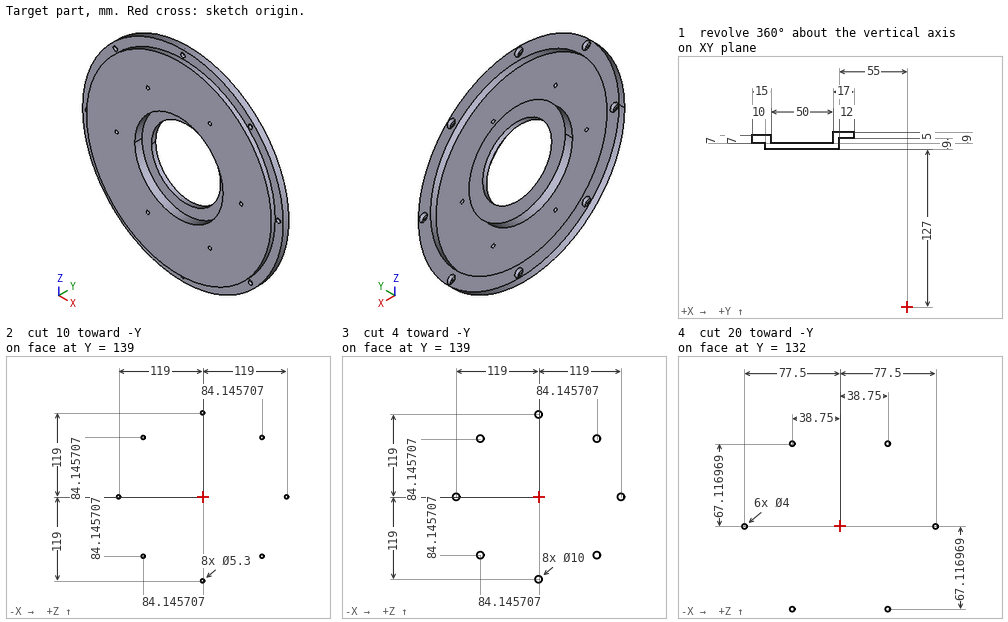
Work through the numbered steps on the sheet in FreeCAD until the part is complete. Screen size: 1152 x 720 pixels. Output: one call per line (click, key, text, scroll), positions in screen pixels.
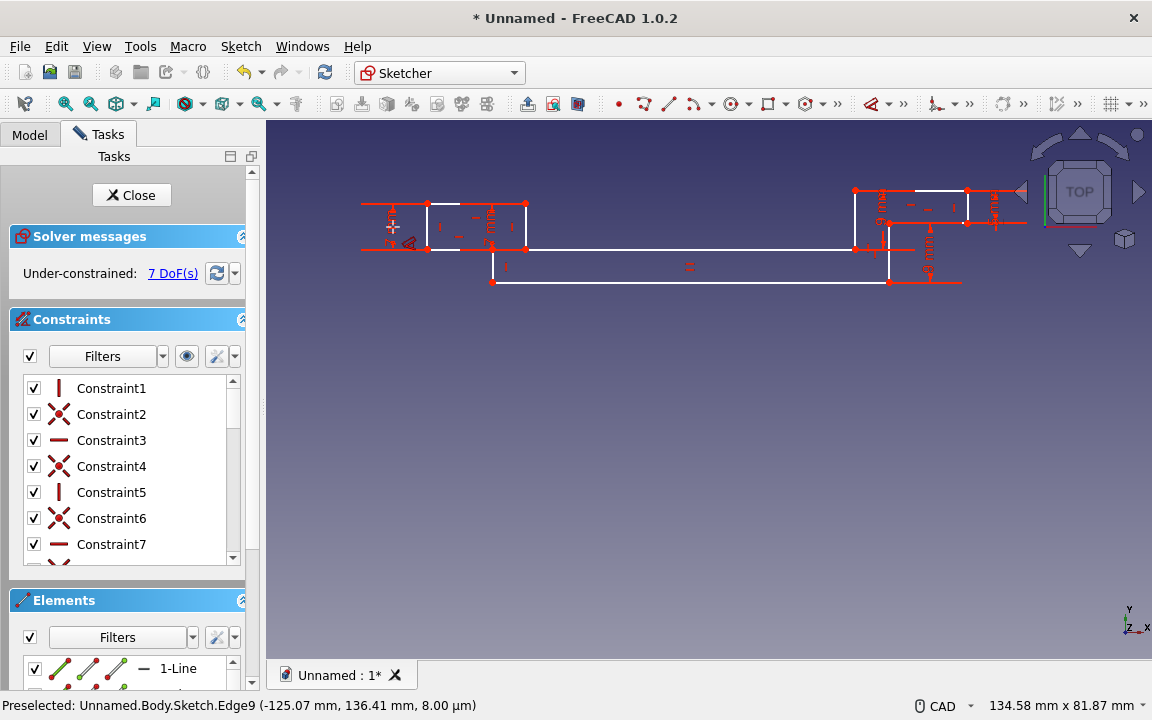
click(913, 223)
click(928, 165)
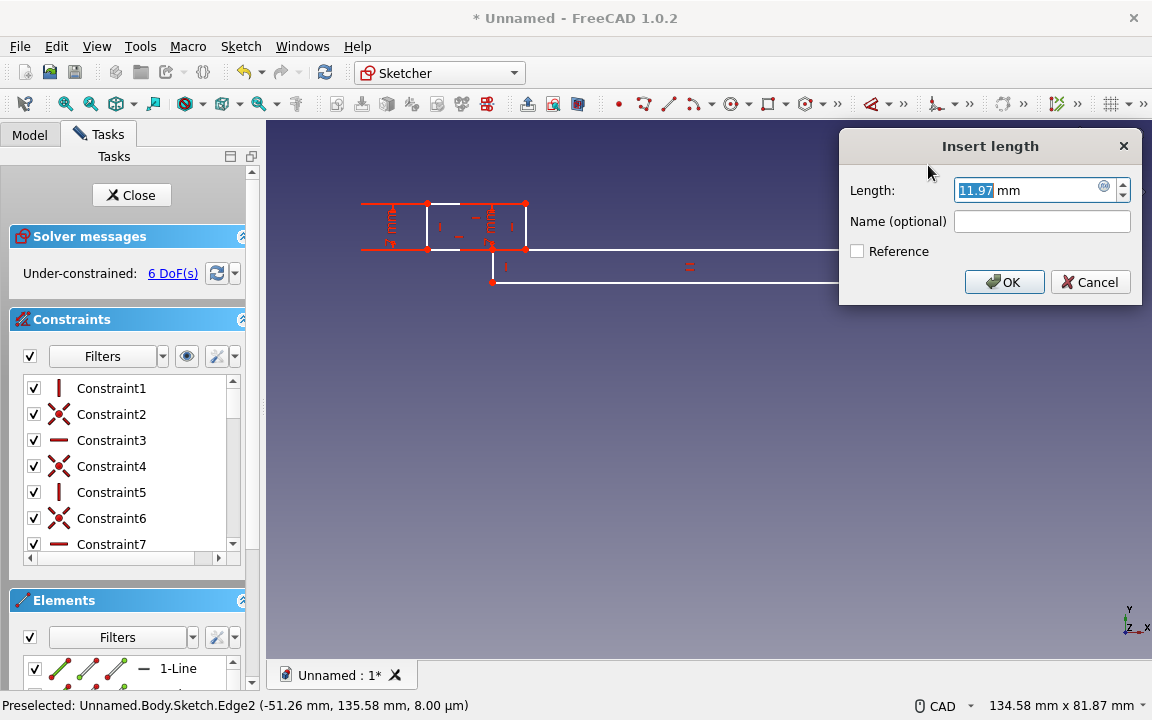
text(12)
key(Return)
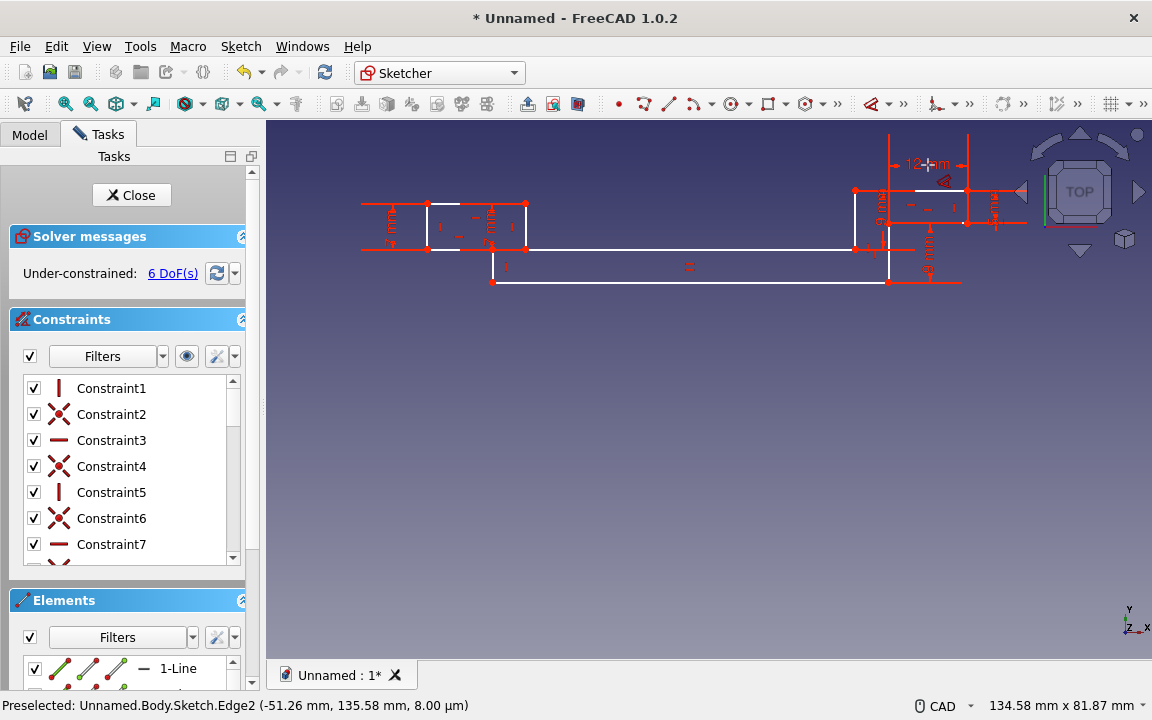
click(934, 191)
click(912, 297)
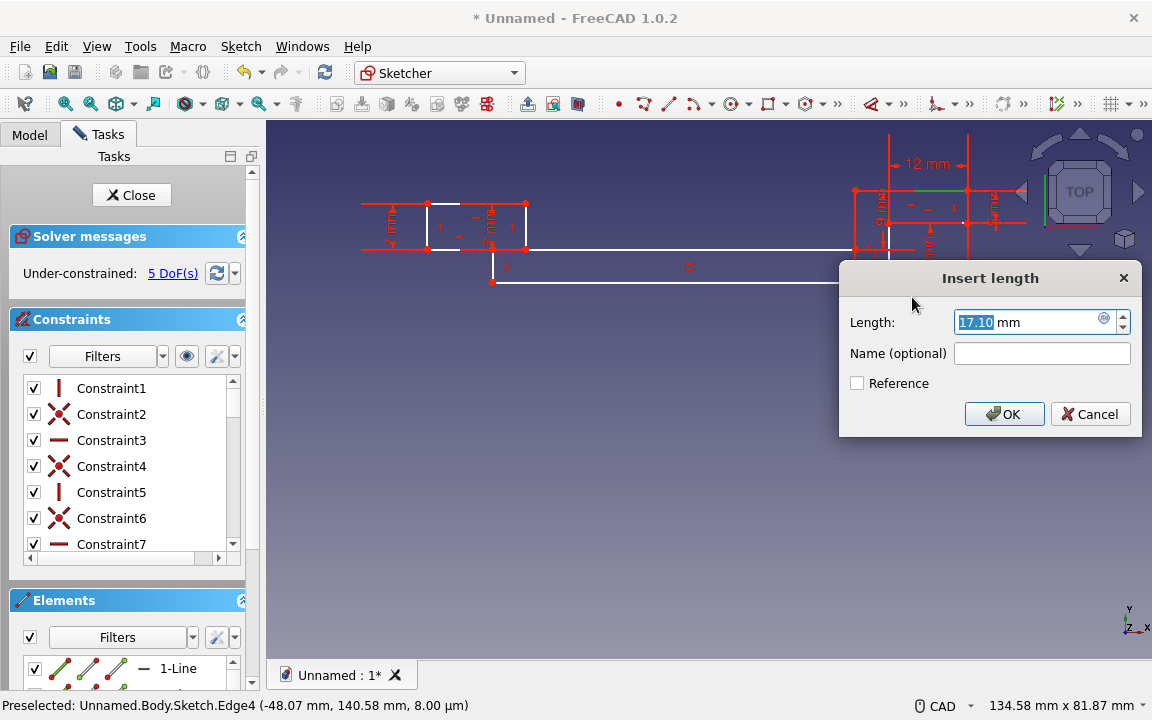
text(17)
key(Return)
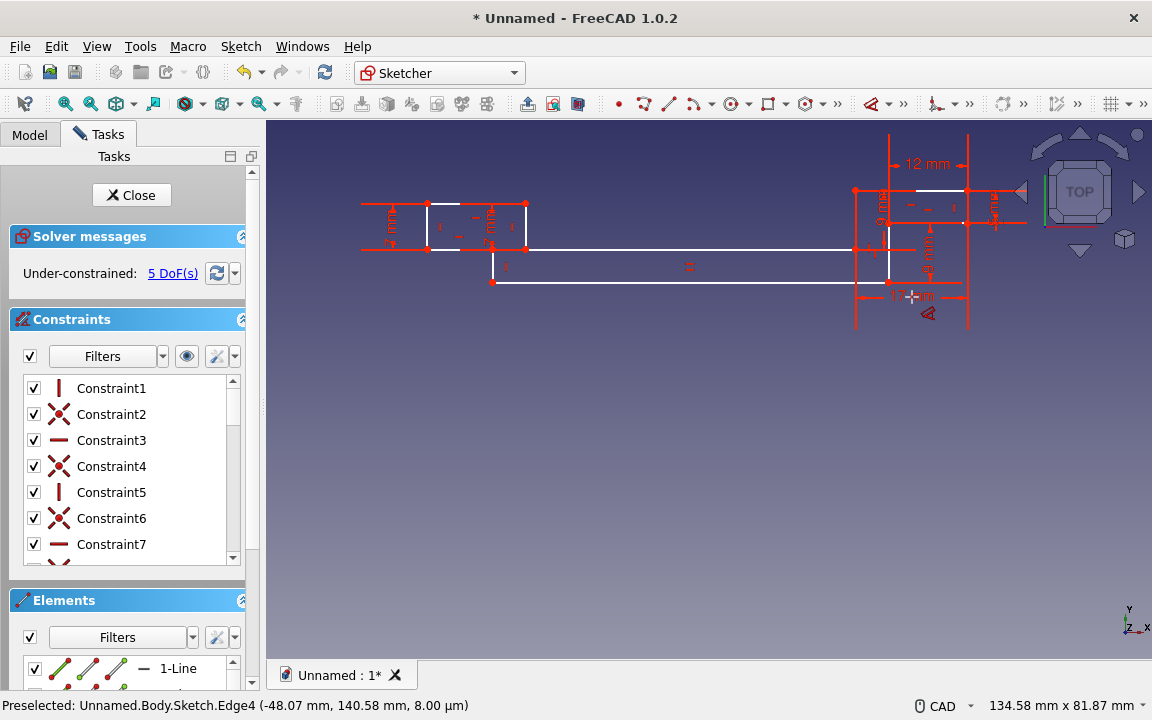
click(757, 250)
click(691, 216)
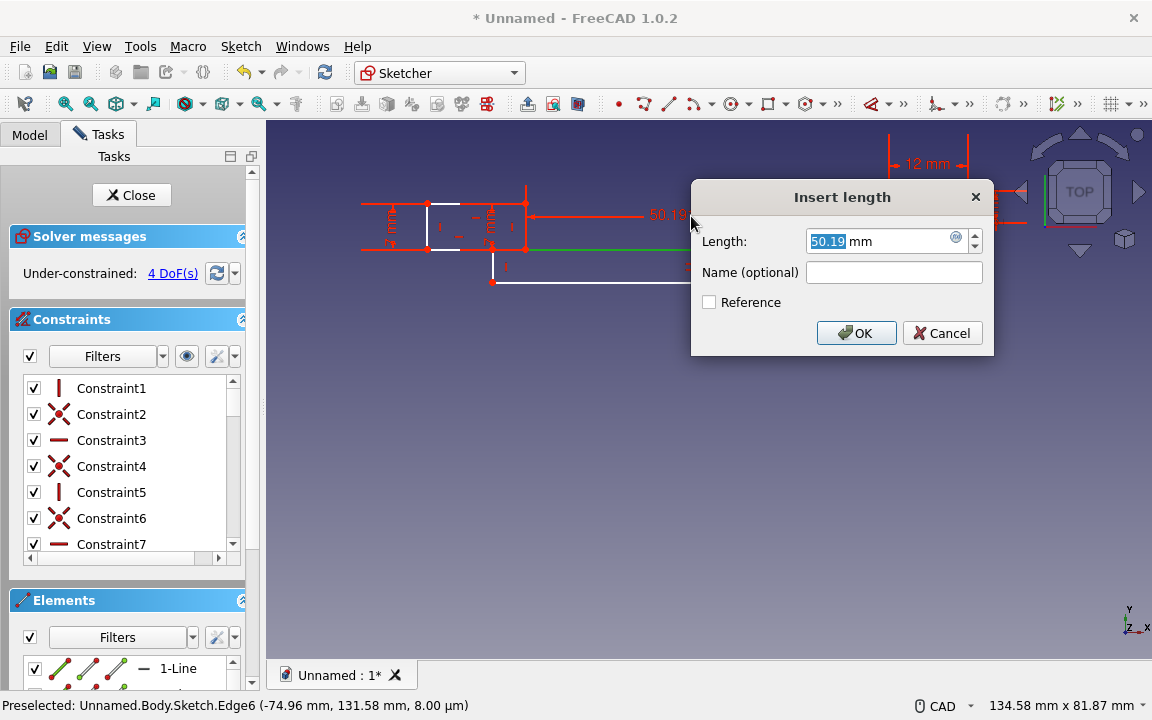
text(50)
key(Return)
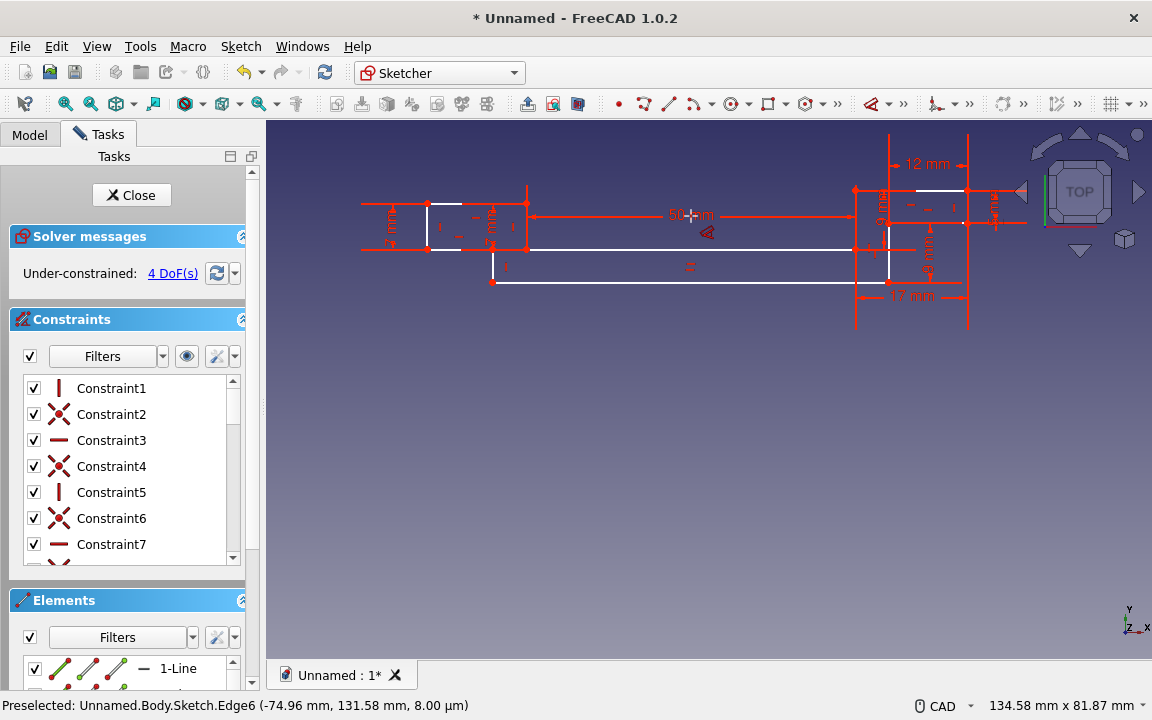
click(497, 204)
click(477, 170)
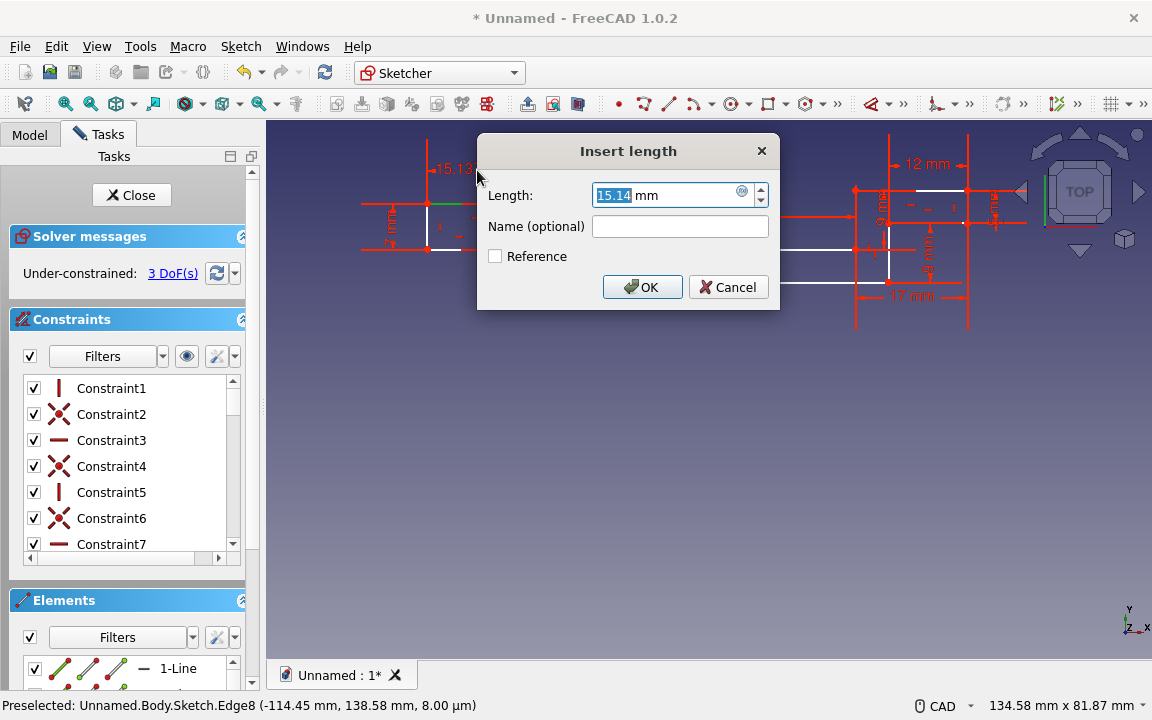
text(15)
key(Return)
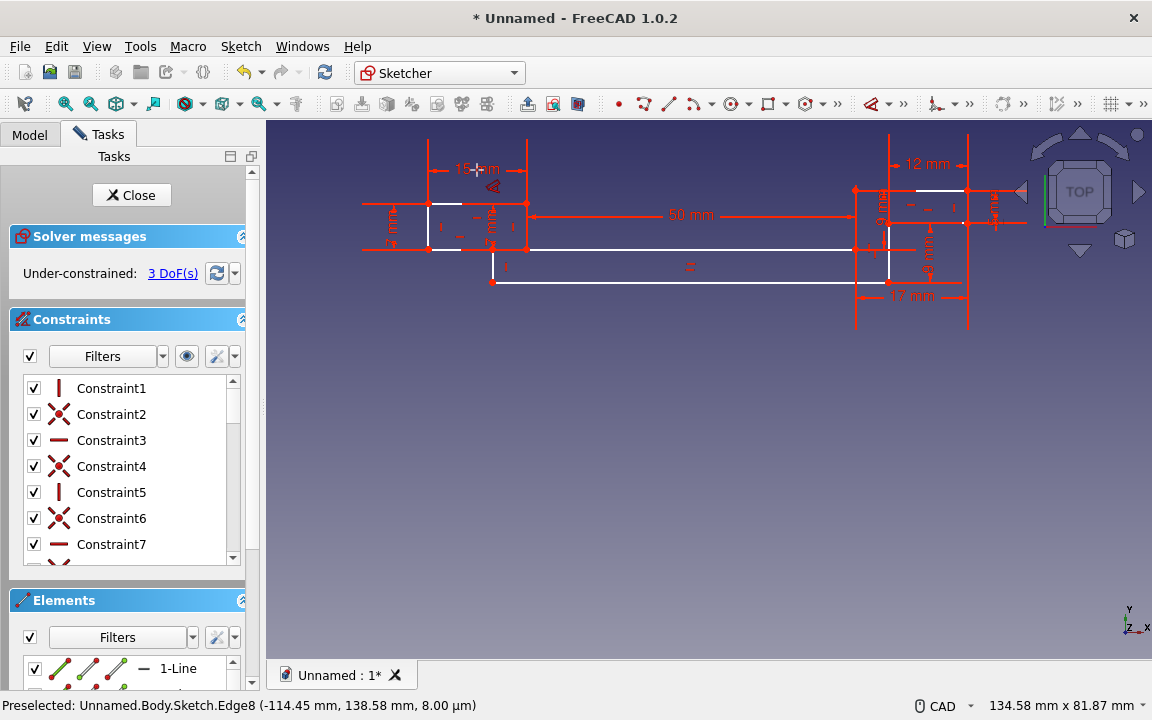
click(447, 250)
click(460, 284)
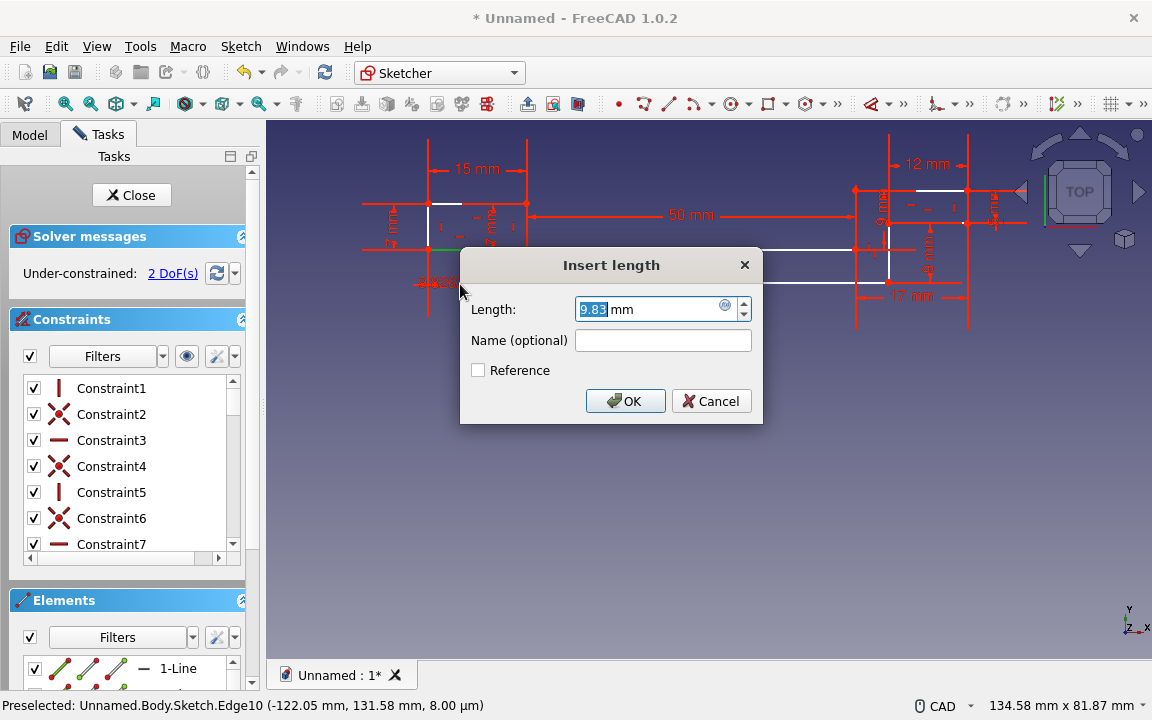
text(10)
key(Return)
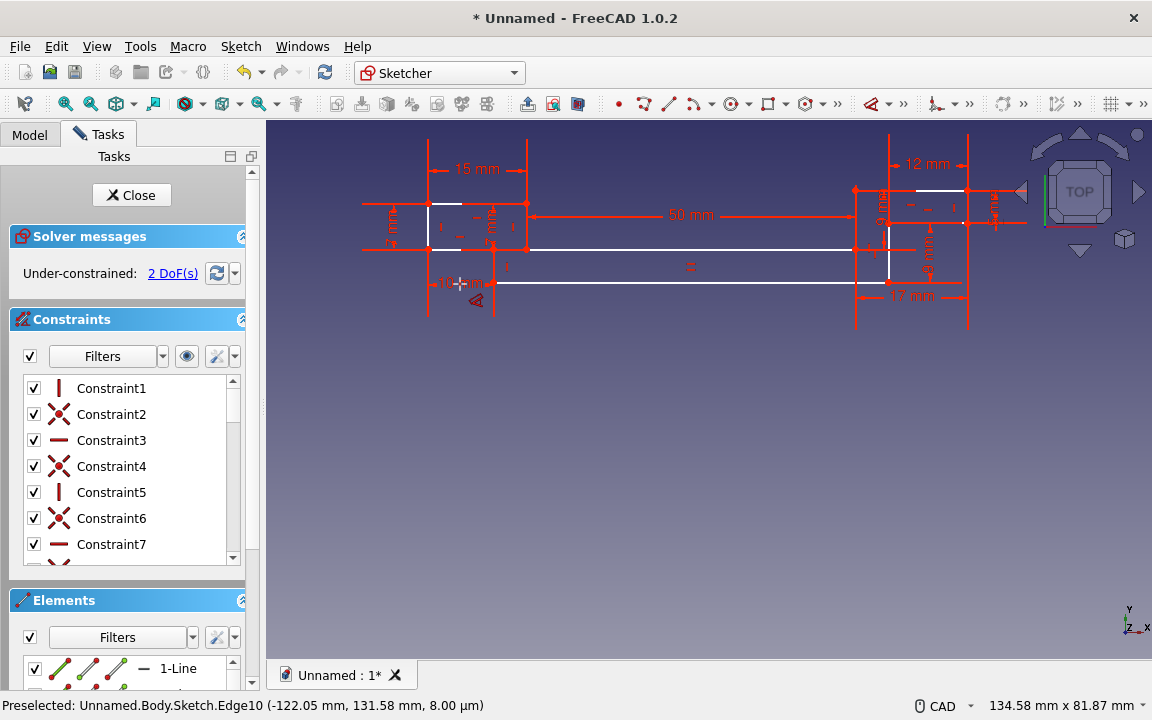
click(889, 283)
click(972, 249)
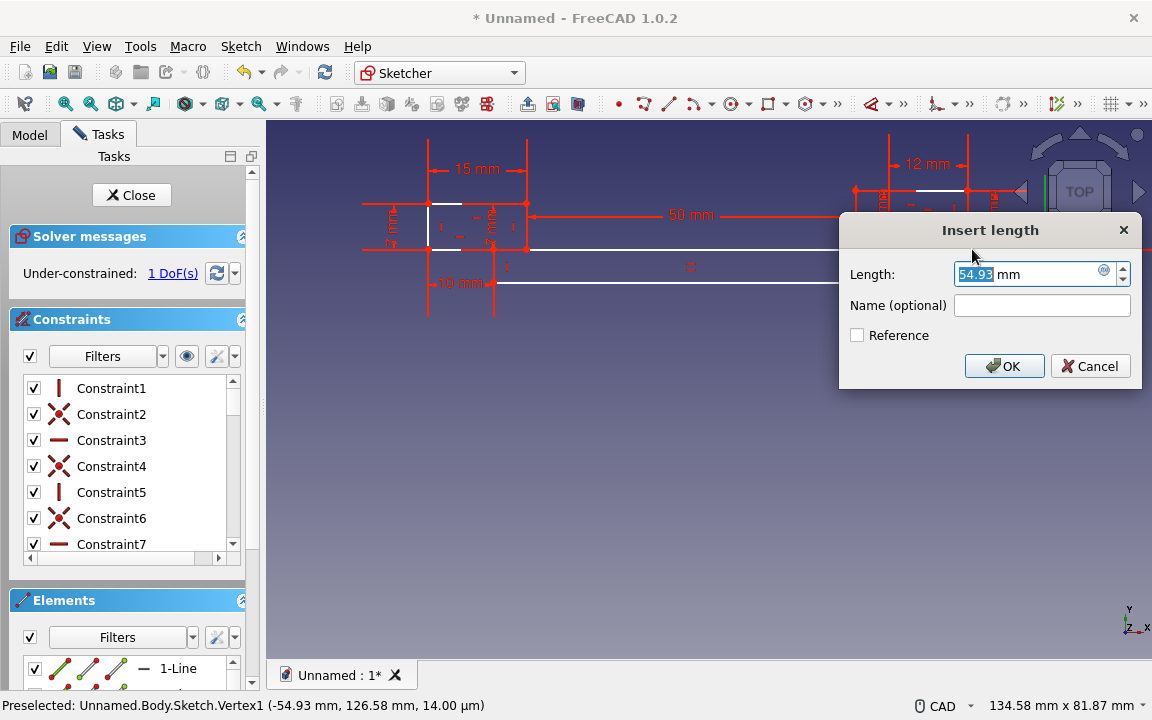
text(55)
key(Return)